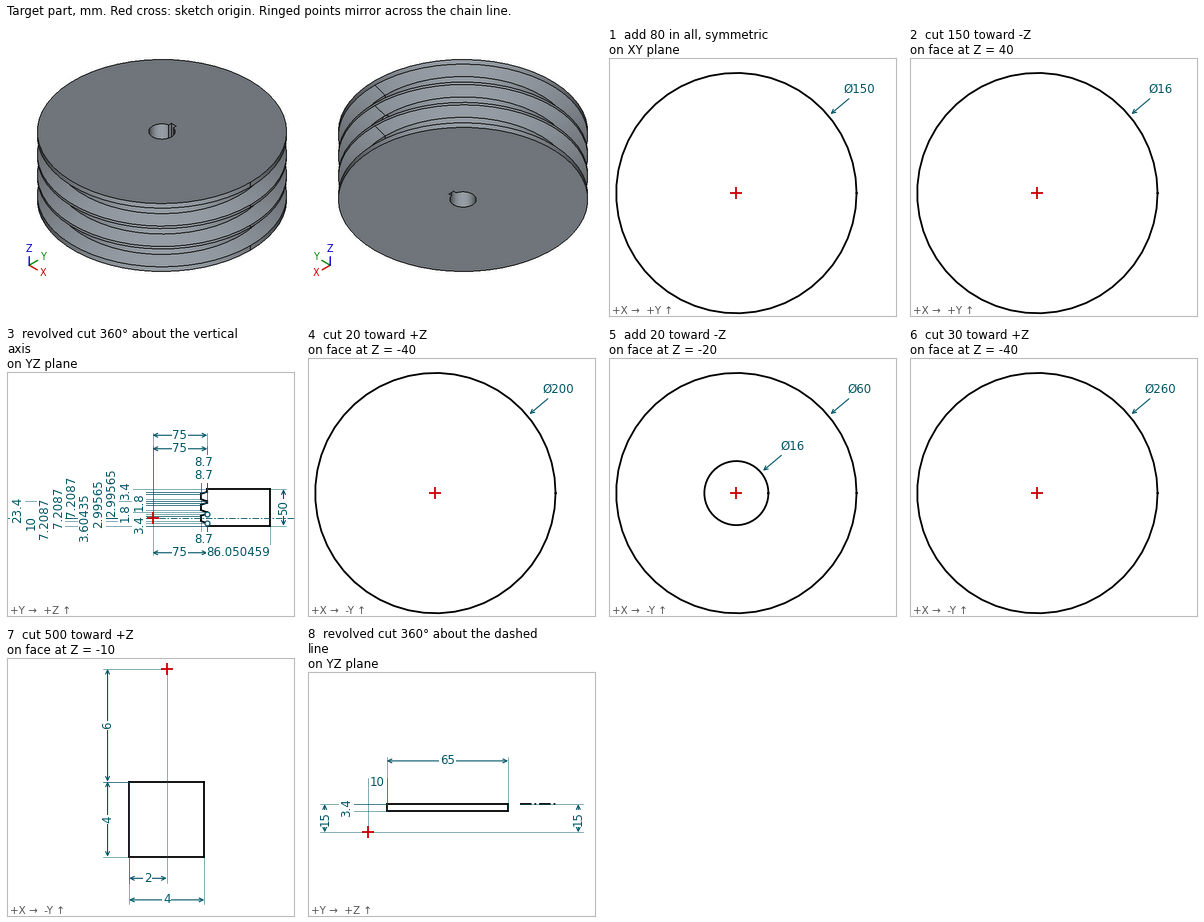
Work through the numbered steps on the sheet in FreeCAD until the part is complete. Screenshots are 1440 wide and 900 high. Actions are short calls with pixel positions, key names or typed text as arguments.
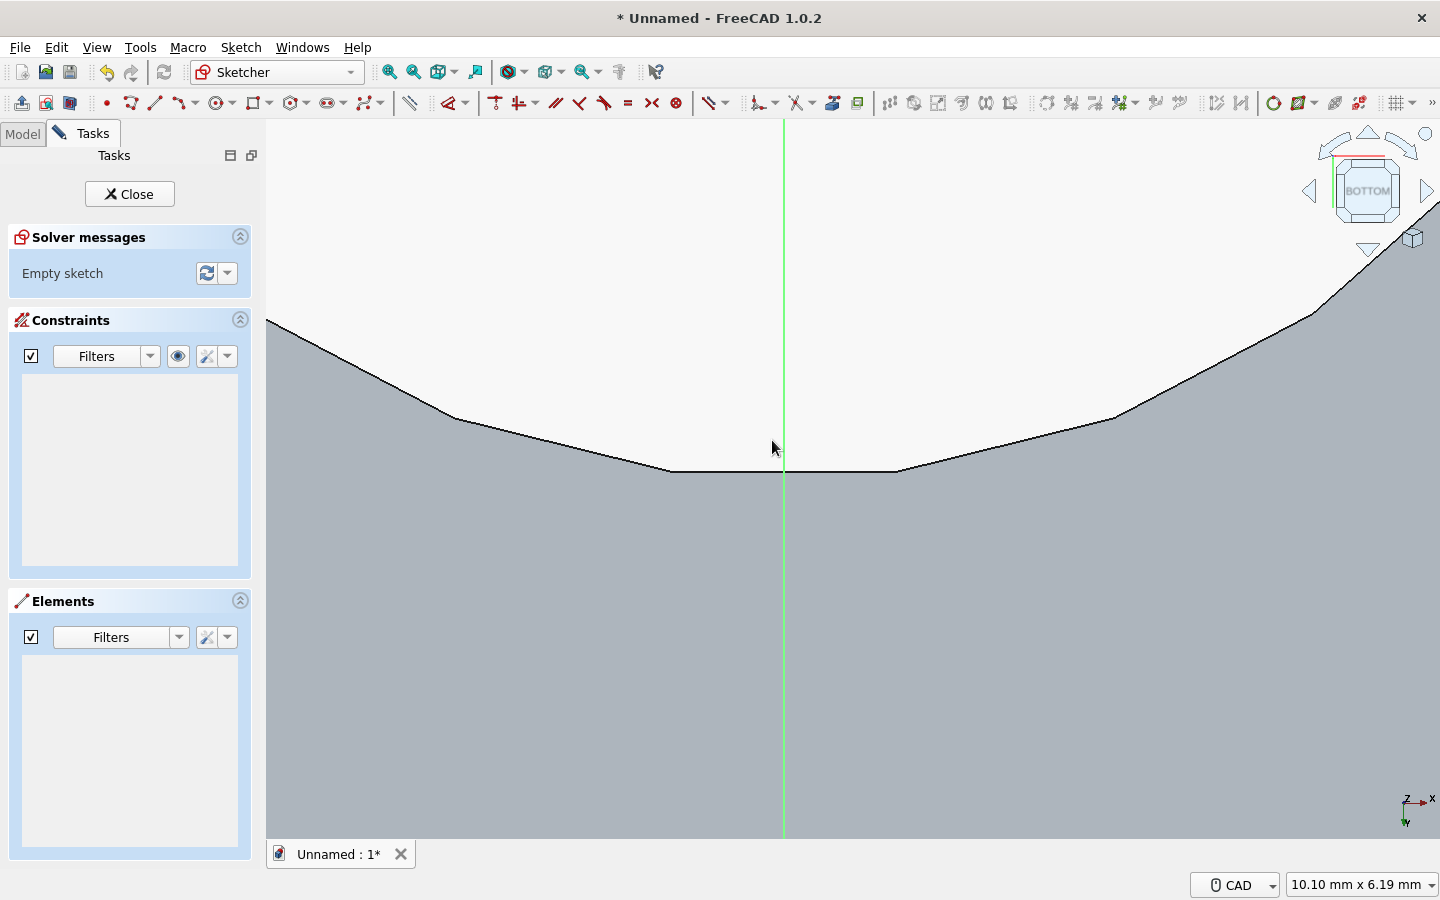
click(254, 104)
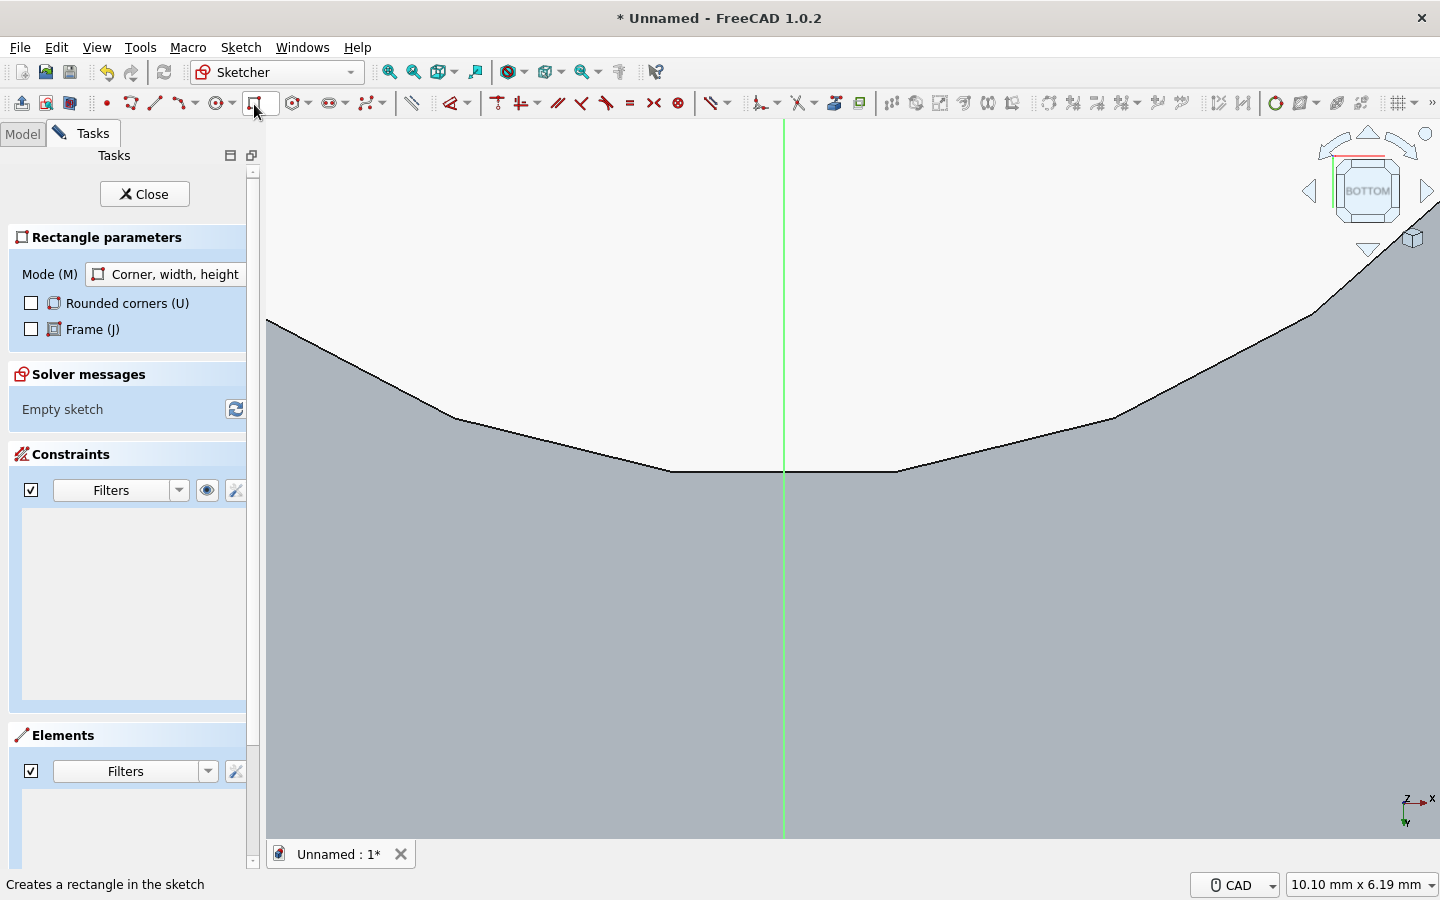
click(552, 246)
click(1017, 711)
key(Escape)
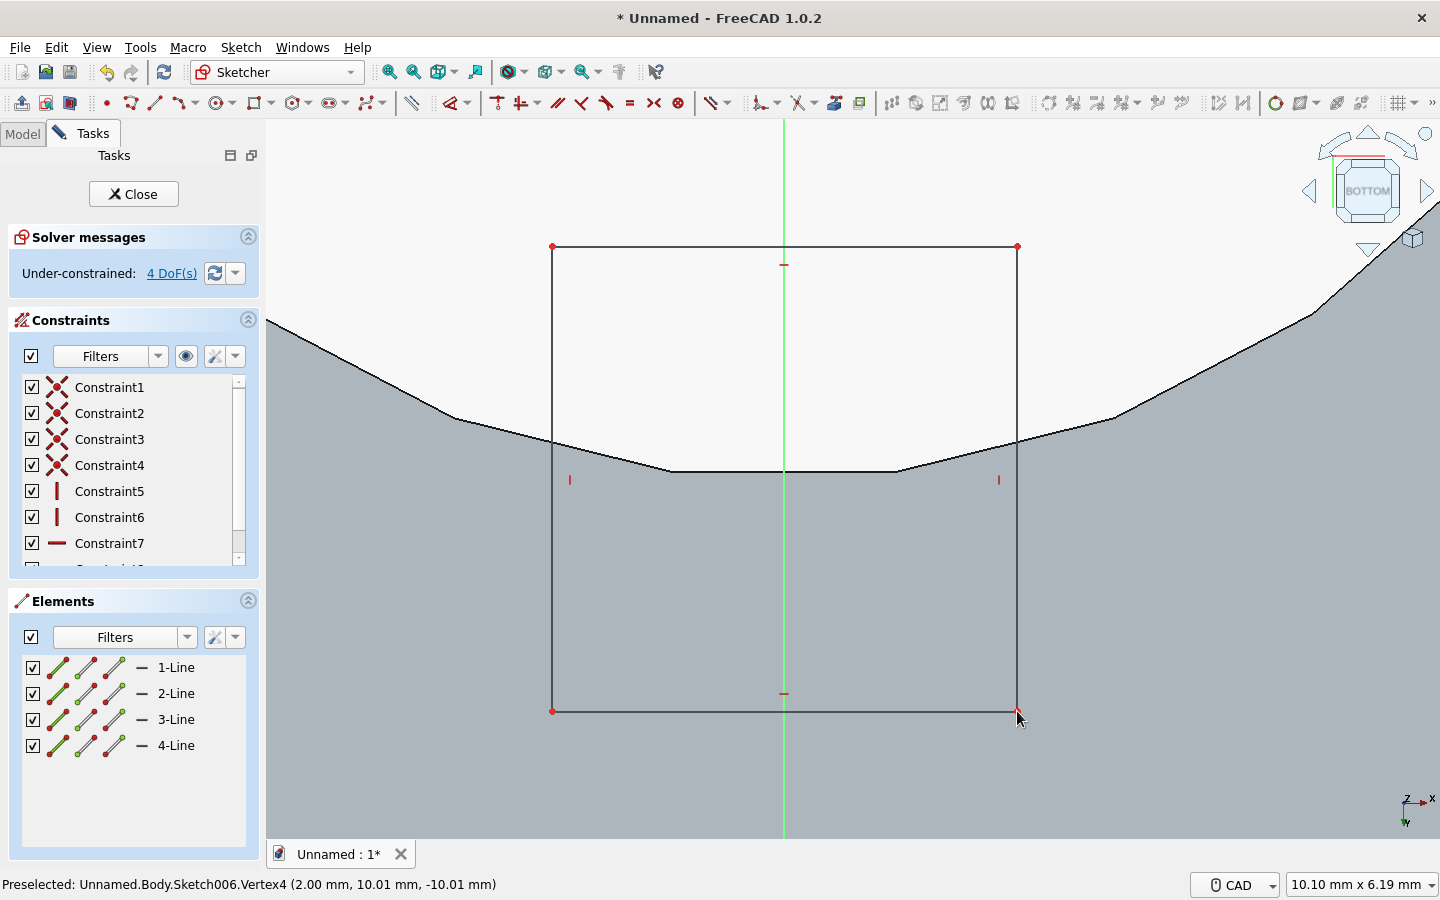
click(450, 104)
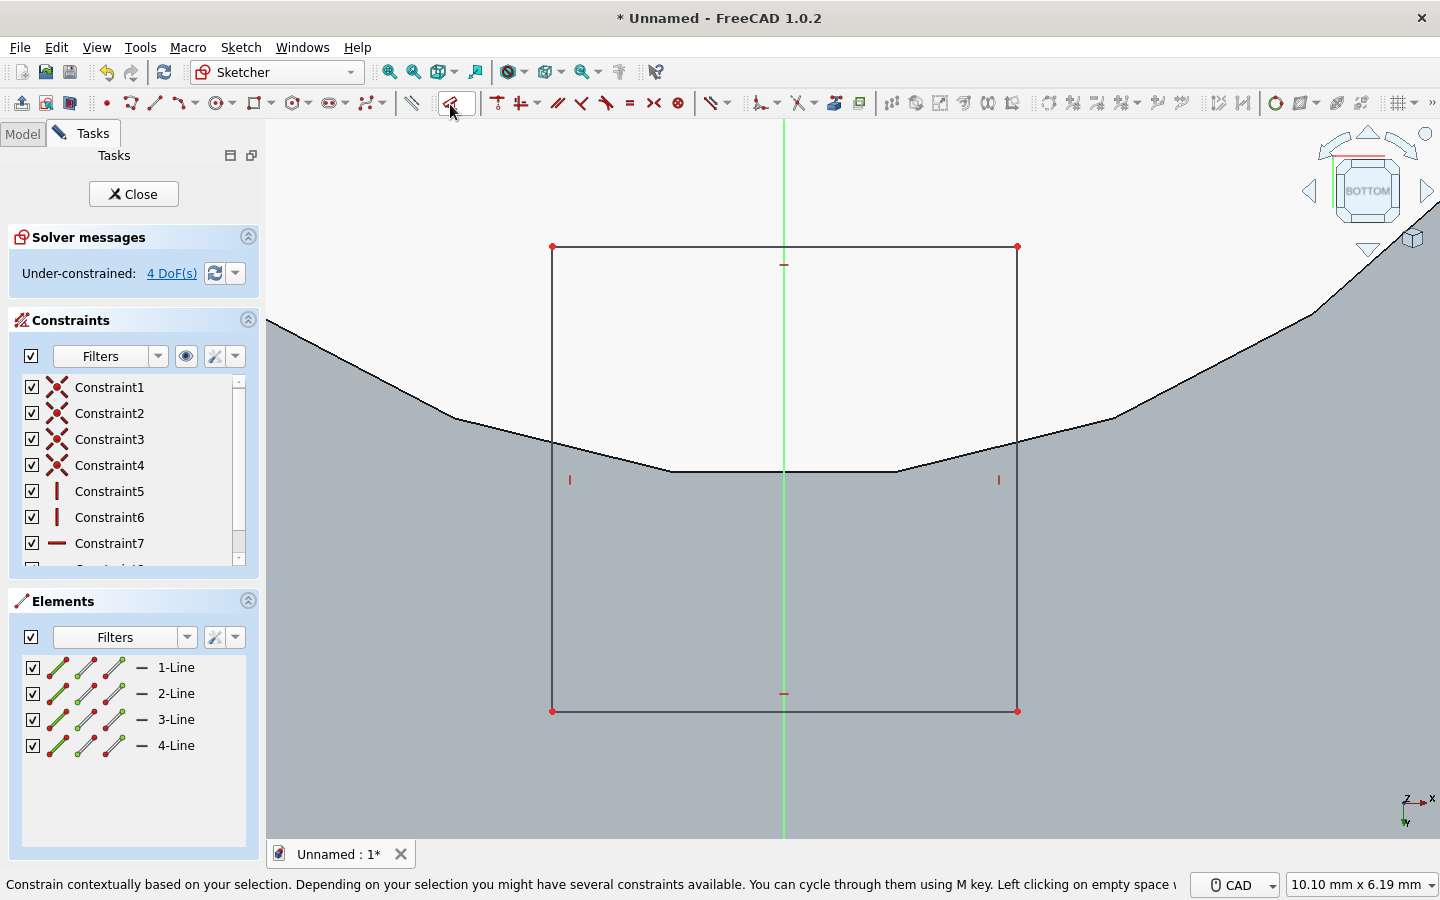
click(552, 386)
click(518, 479)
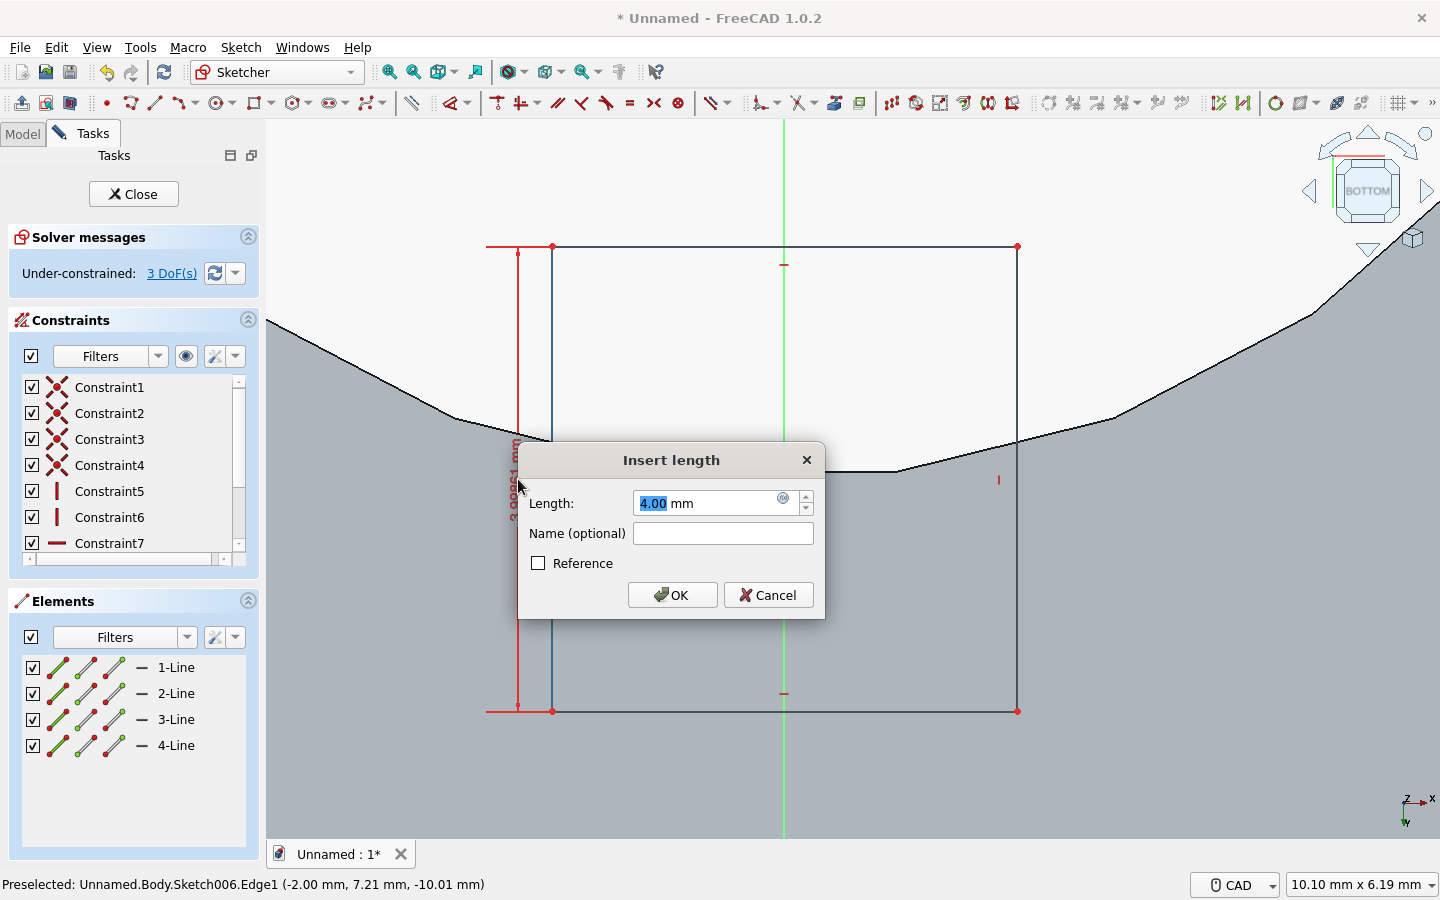
text(4)
key(Return)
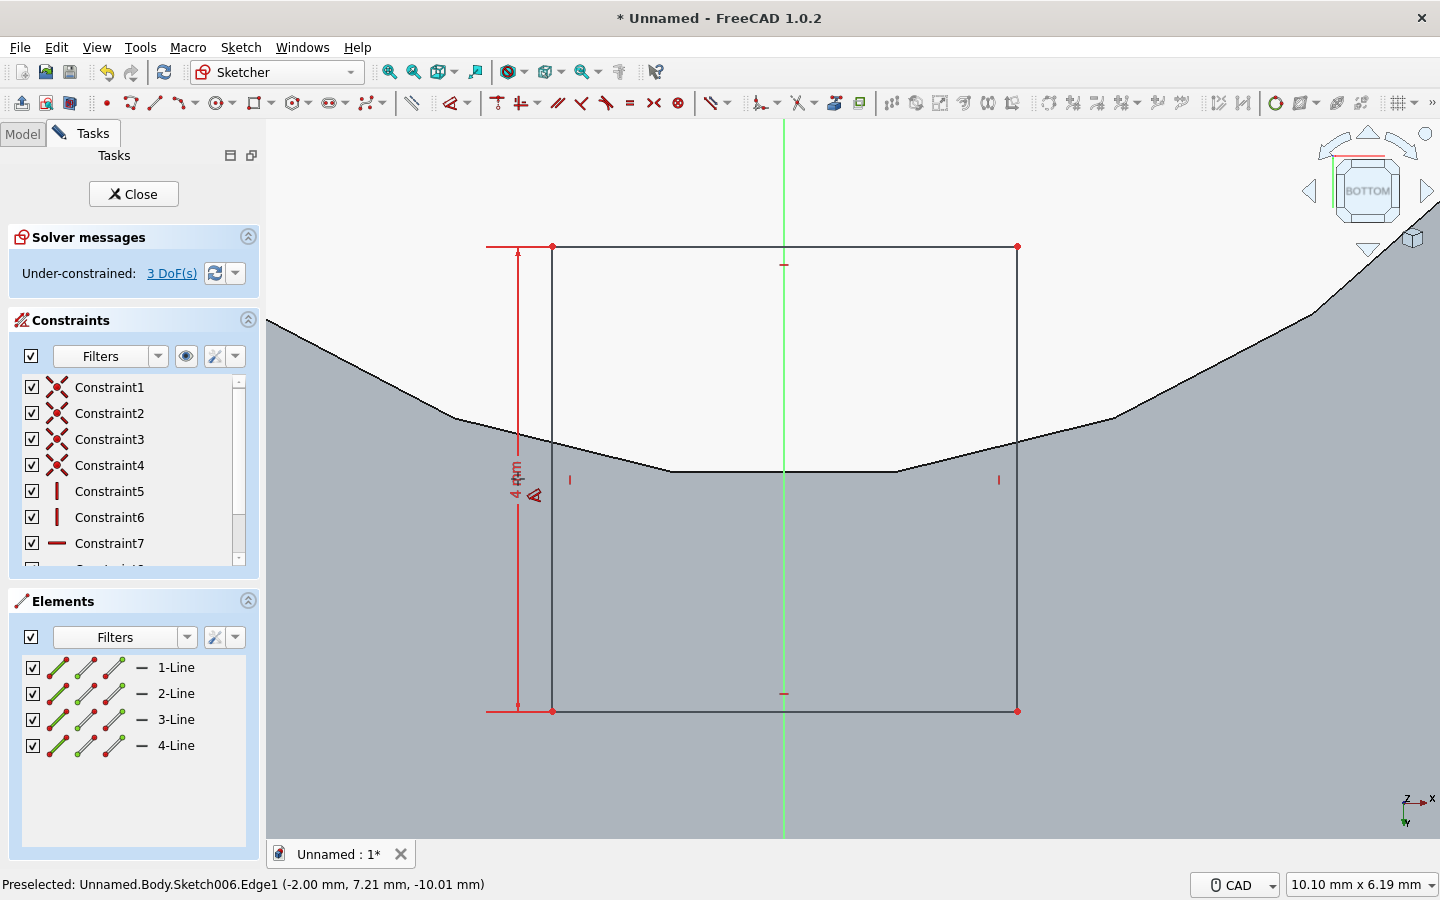
click(692, 712)
click(678, 746)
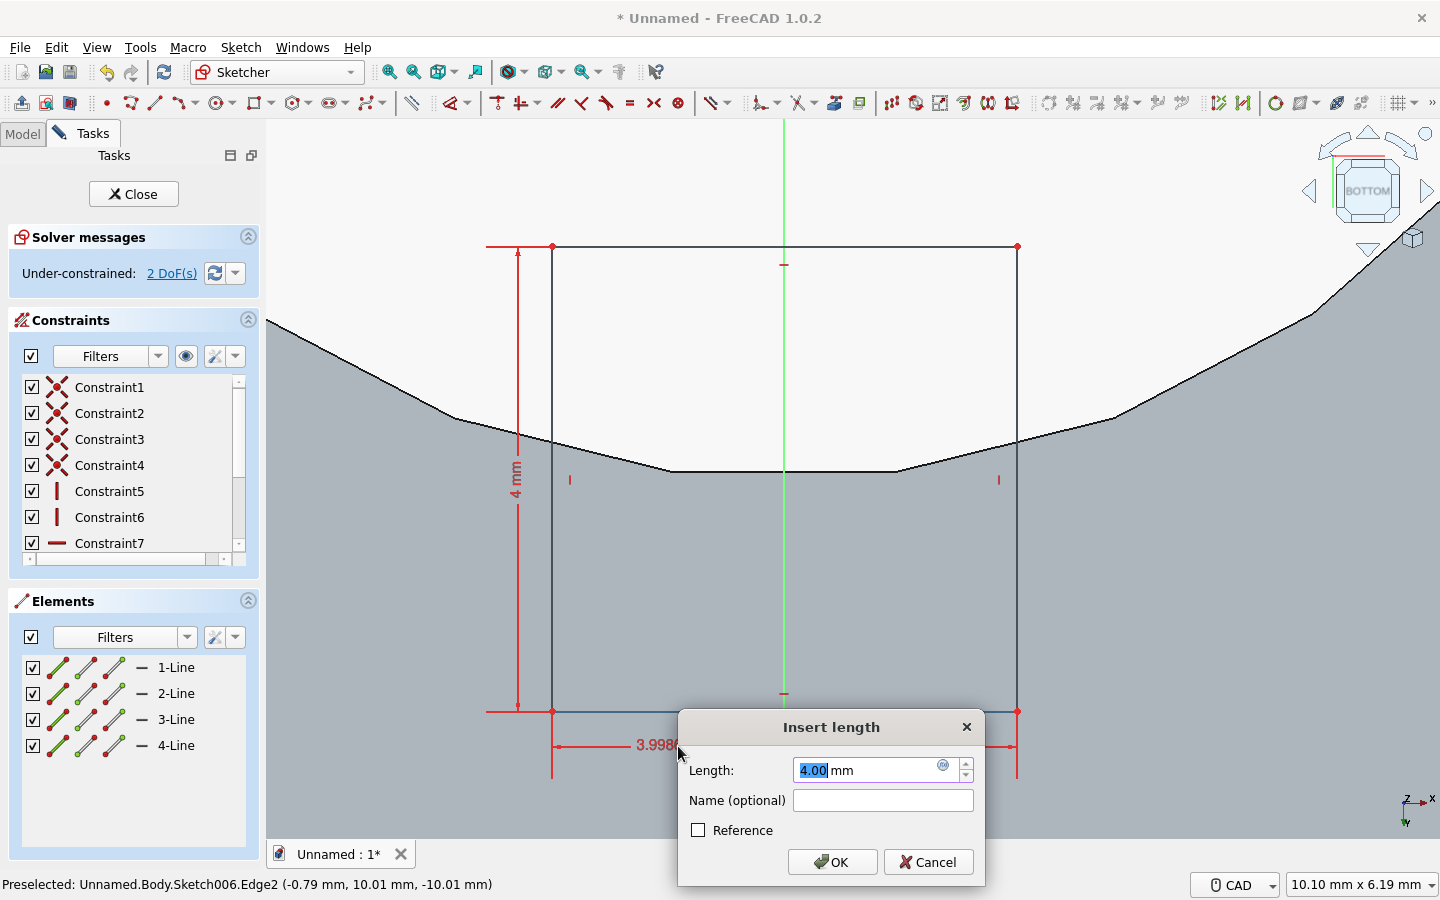
text(4)
key(Return)